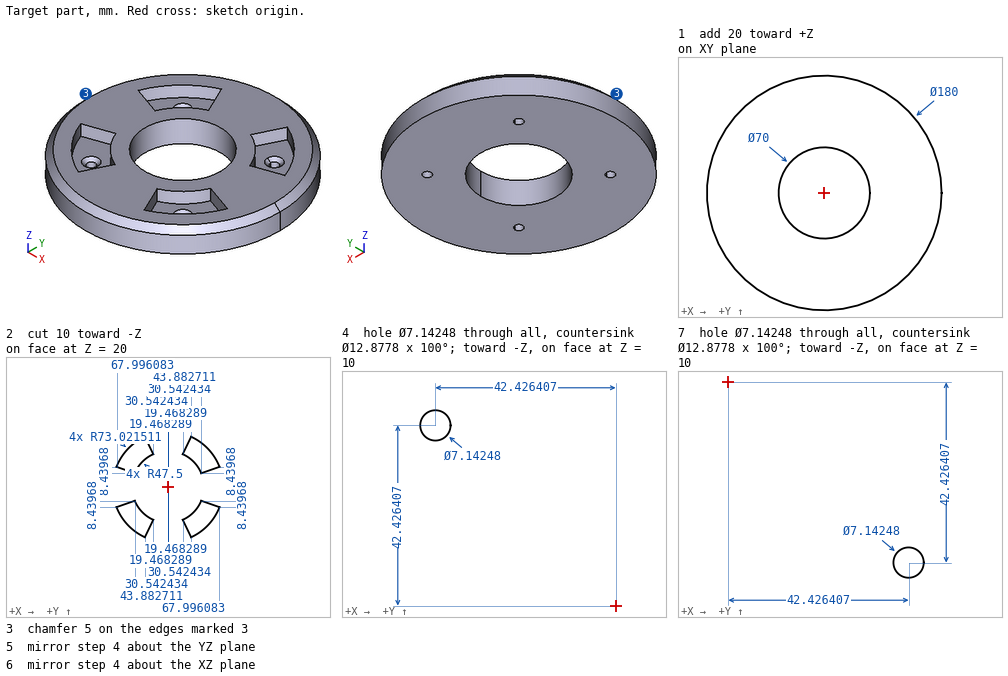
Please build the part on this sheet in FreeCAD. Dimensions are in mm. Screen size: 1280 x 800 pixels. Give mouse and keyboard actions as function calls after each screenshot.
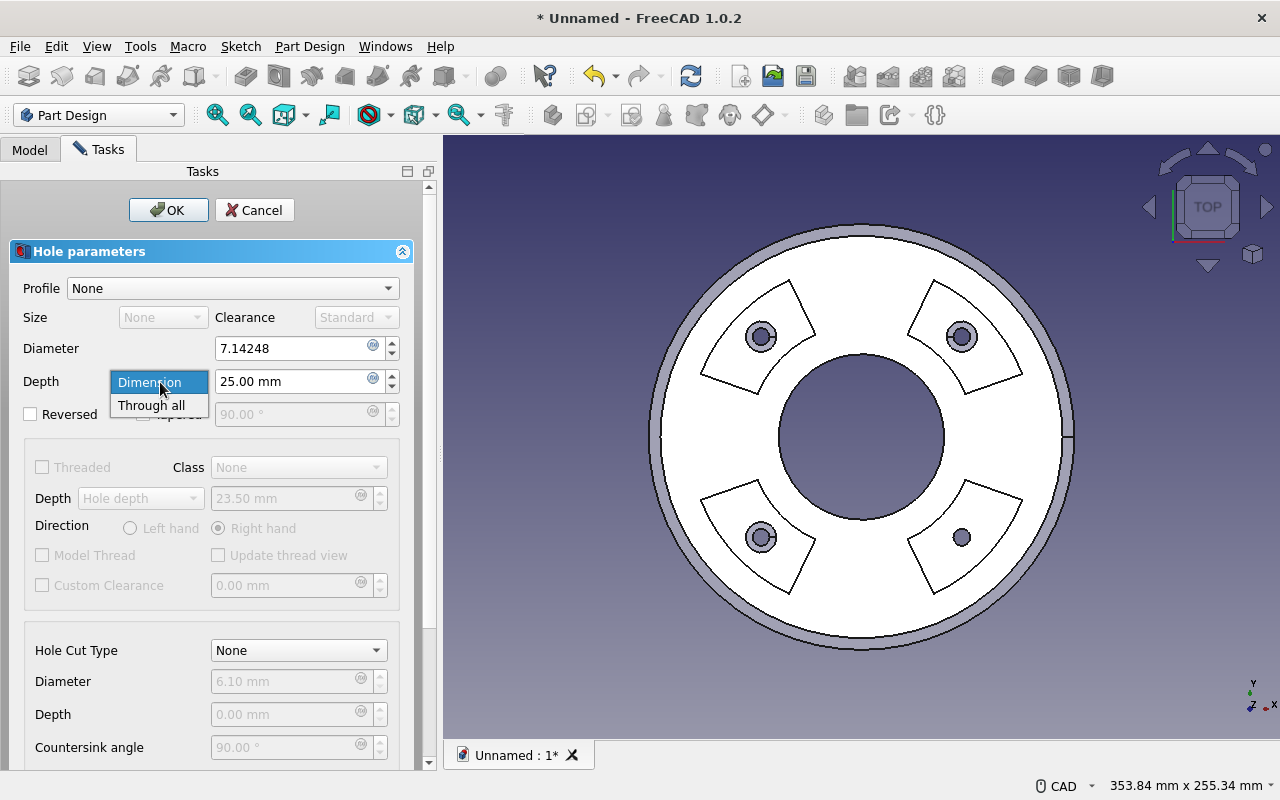
click(158, 406)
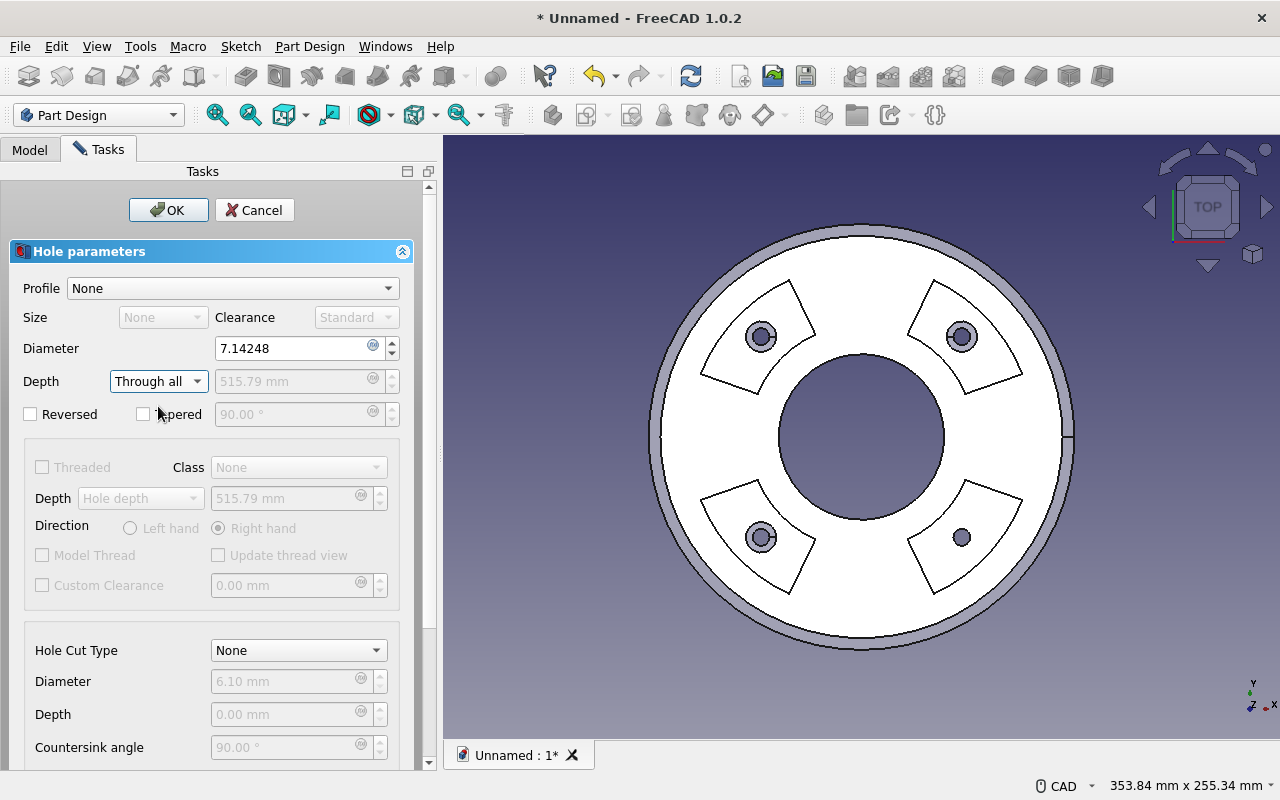
click(300, 650)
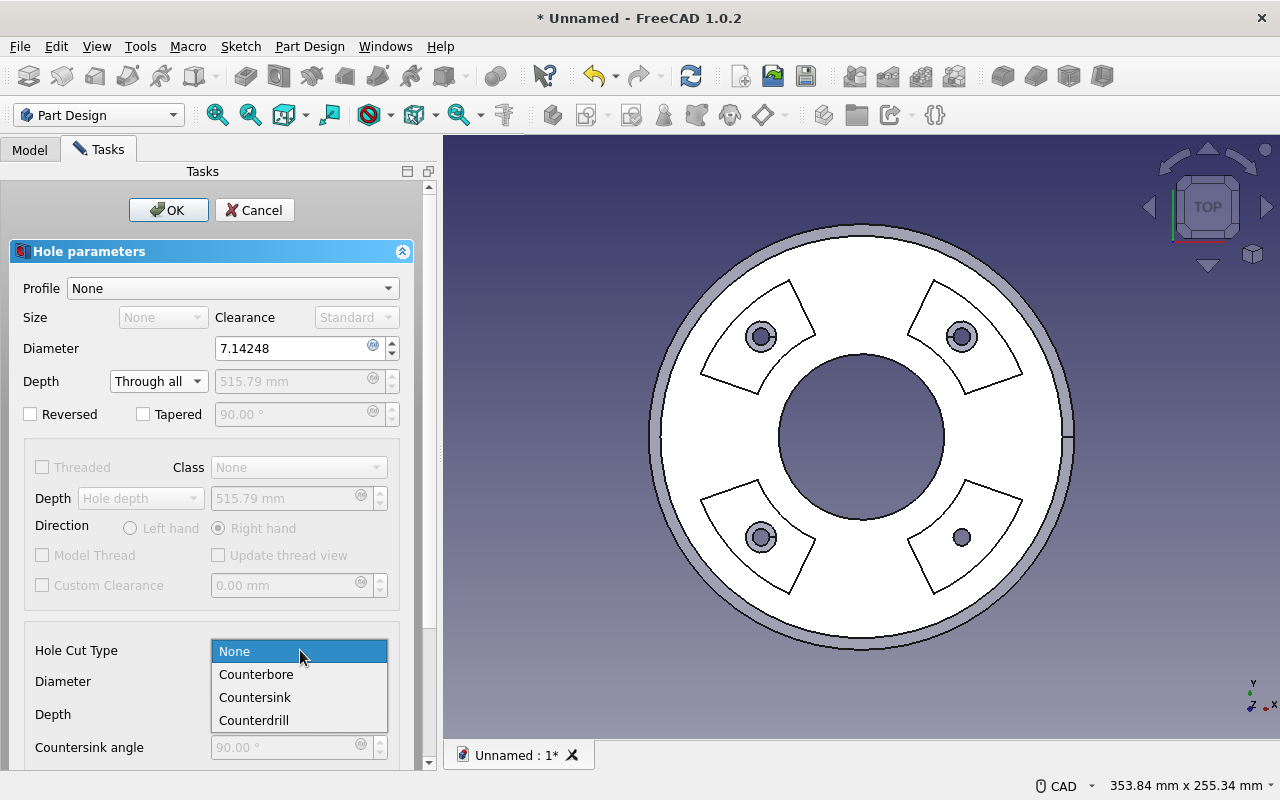
click(298, 698)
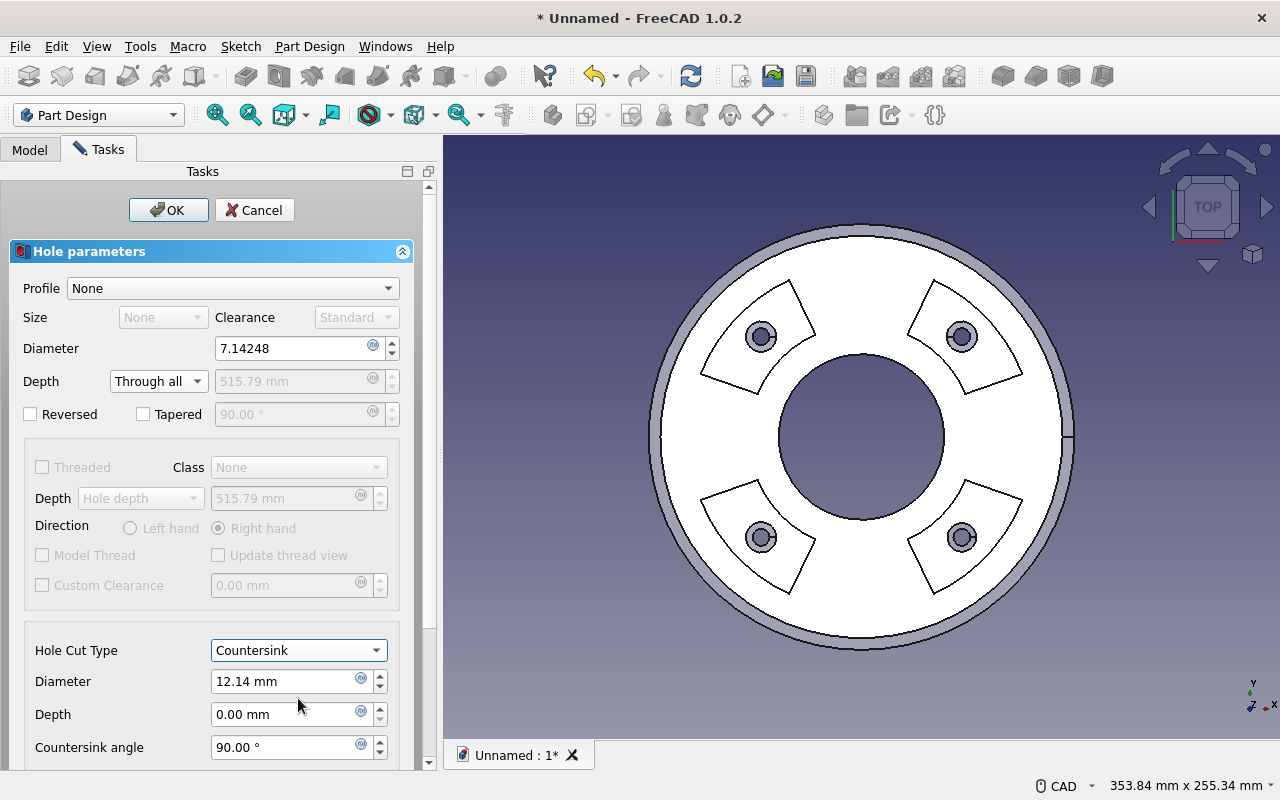
triple_click(292, 748)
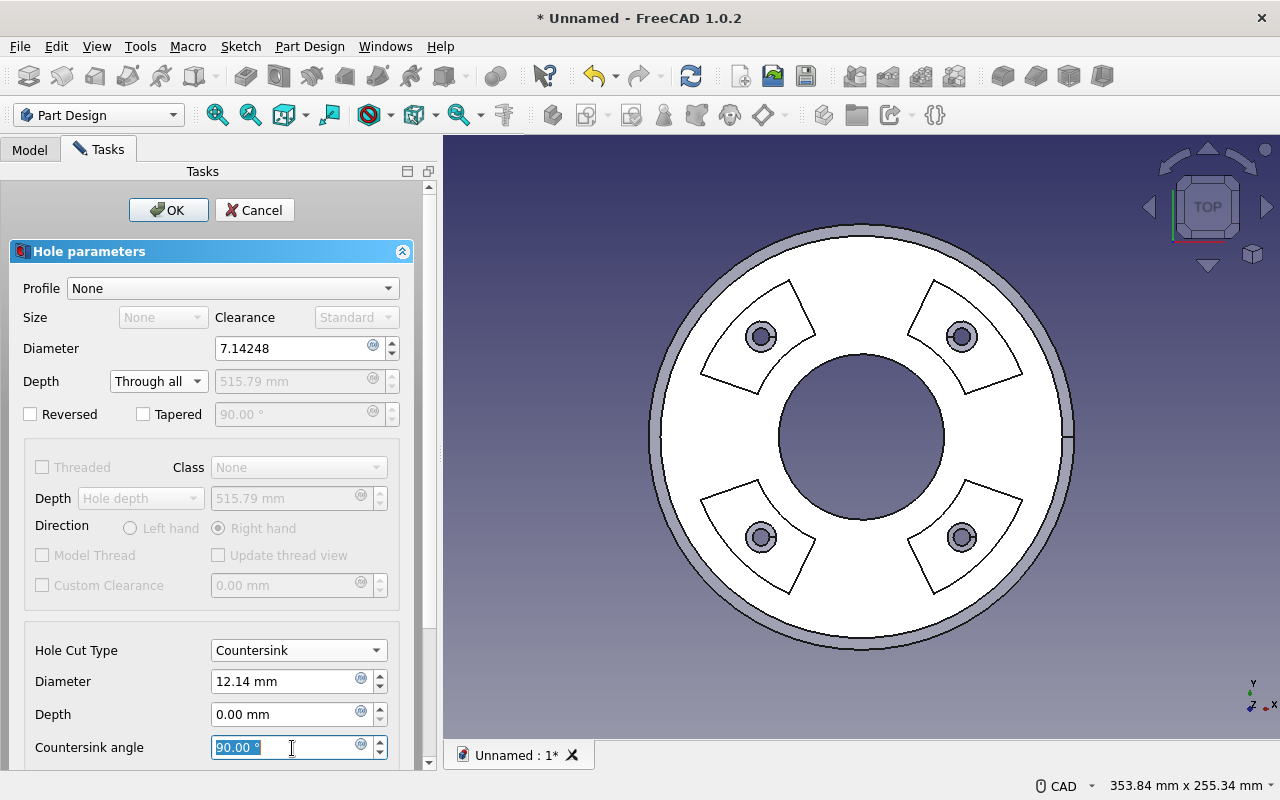
text(100)
key(Tab)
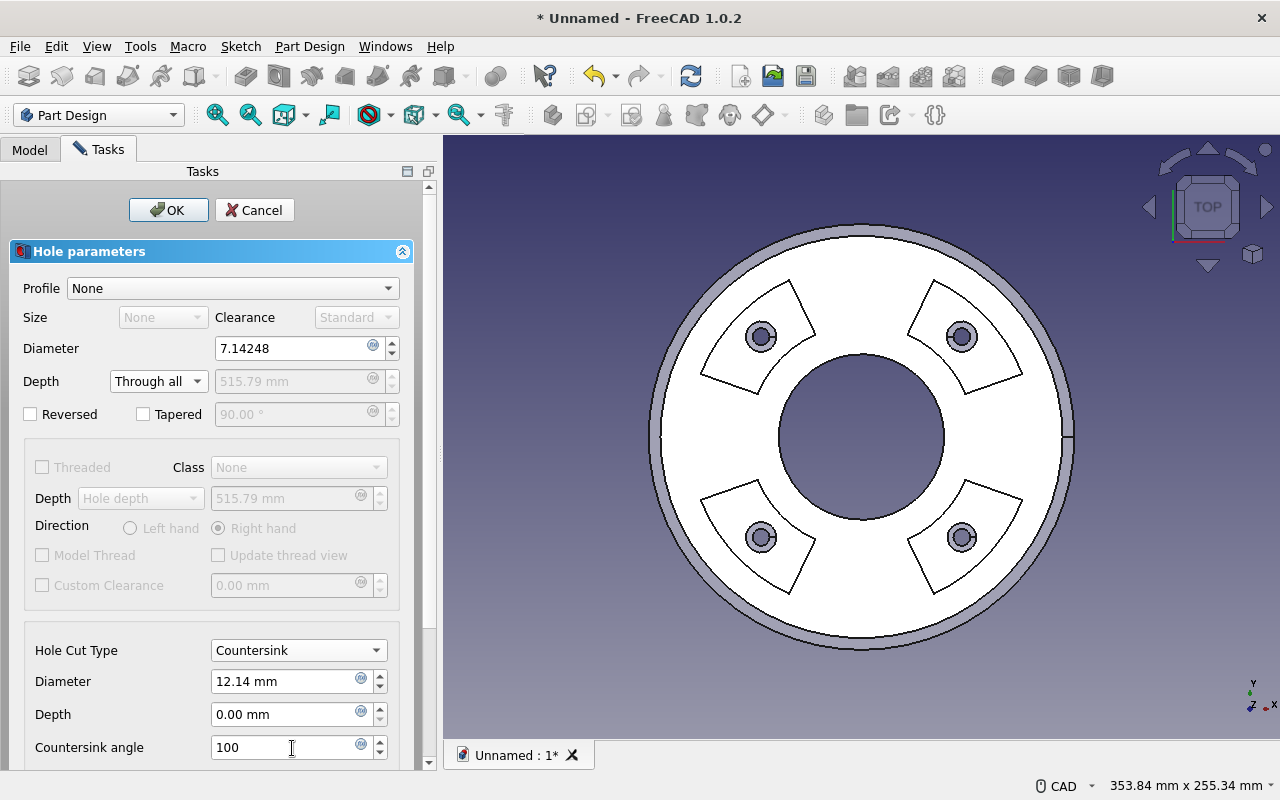
triple_click(292, 682)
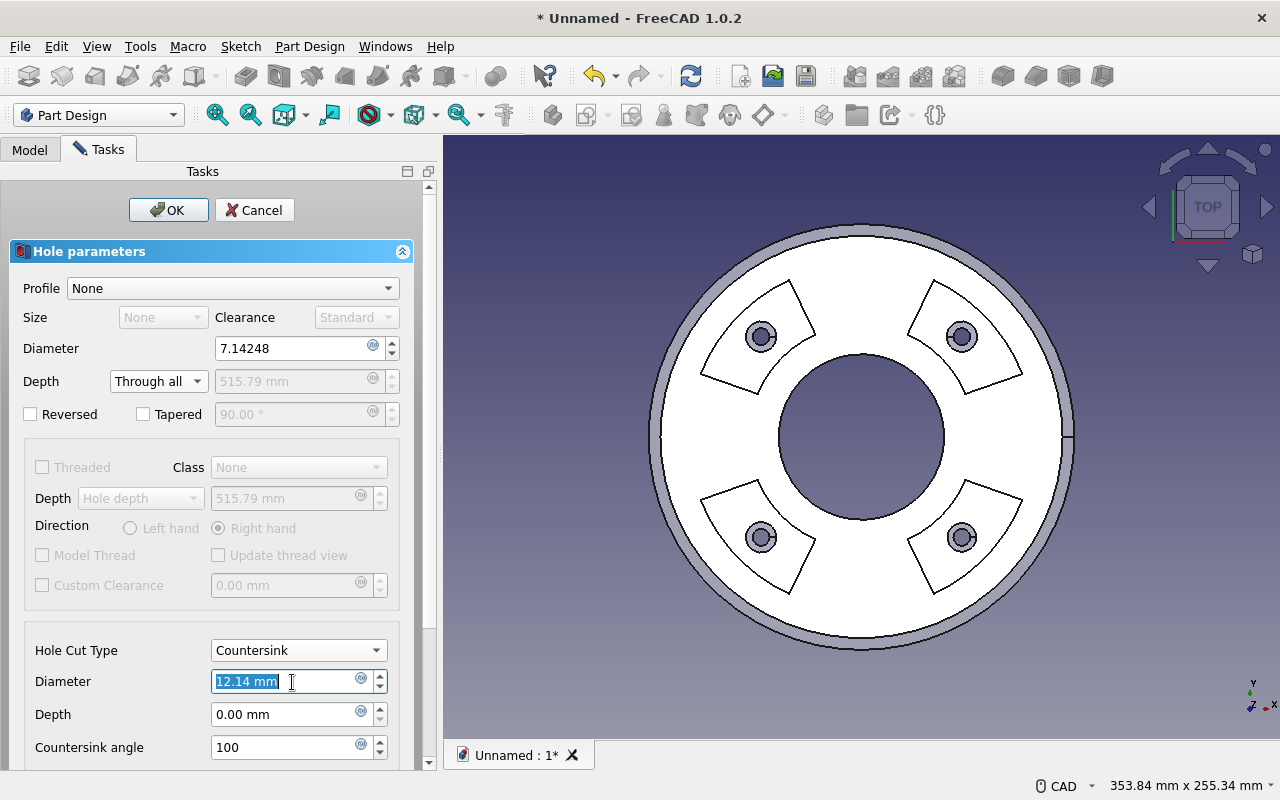
text(12.8778)
key(Tab)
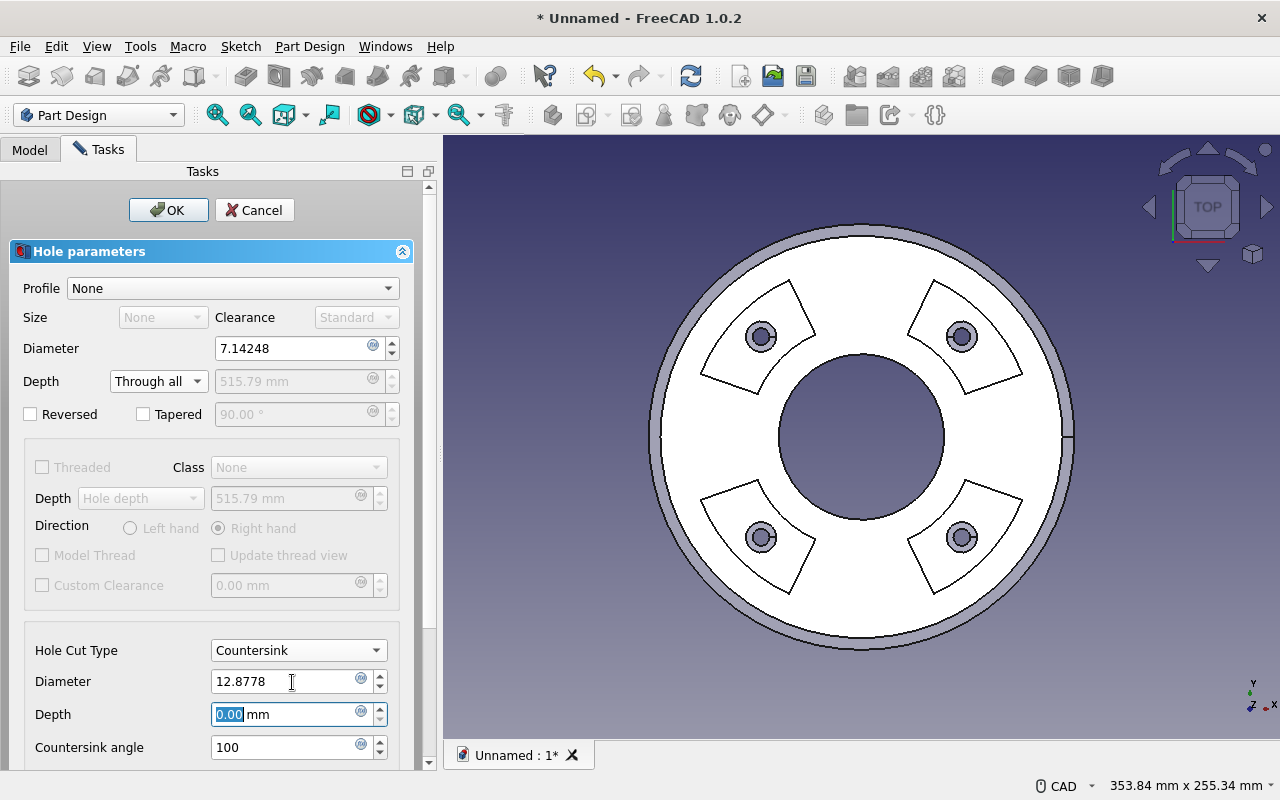
click(169, 210)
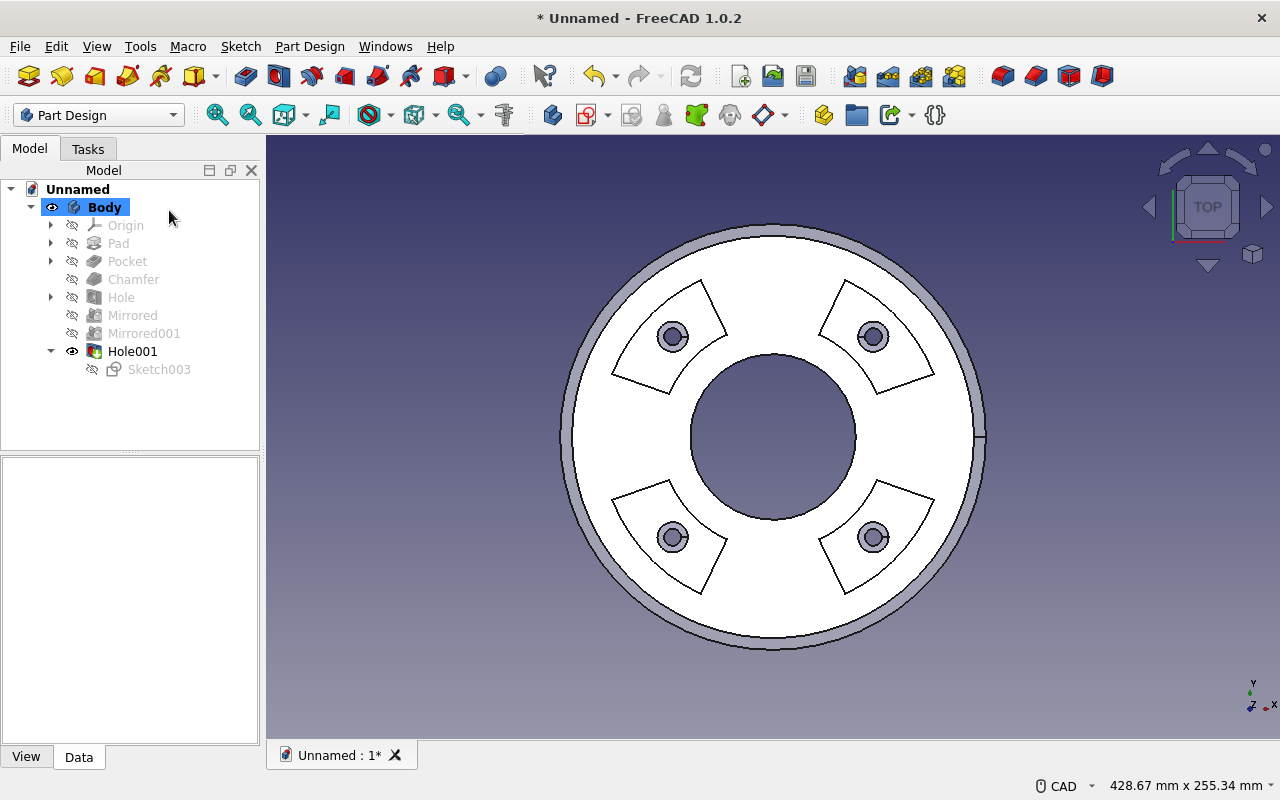
key(0)